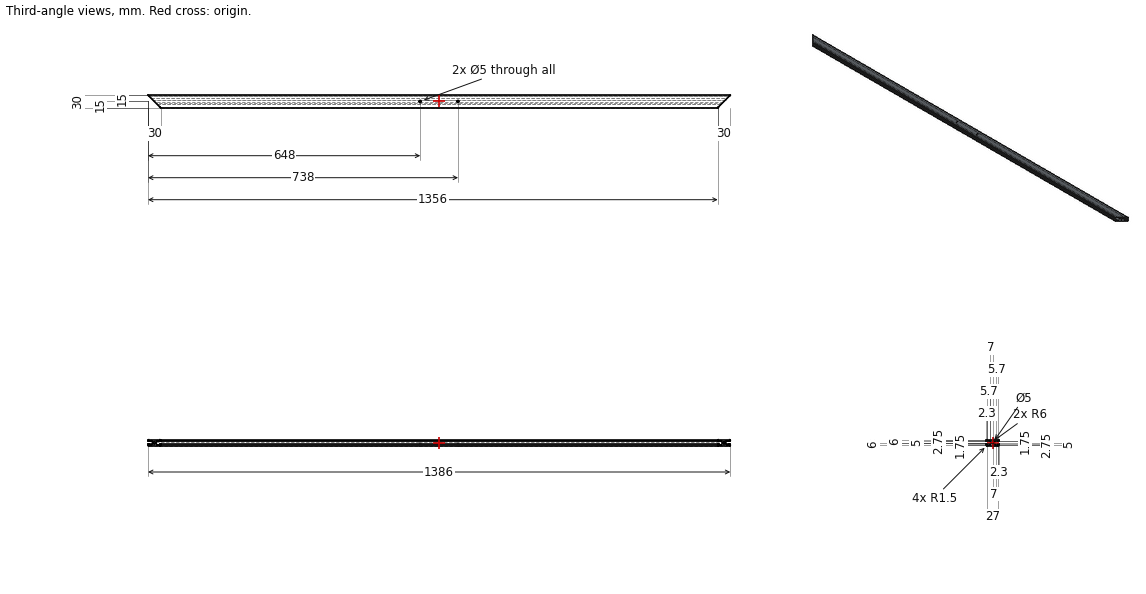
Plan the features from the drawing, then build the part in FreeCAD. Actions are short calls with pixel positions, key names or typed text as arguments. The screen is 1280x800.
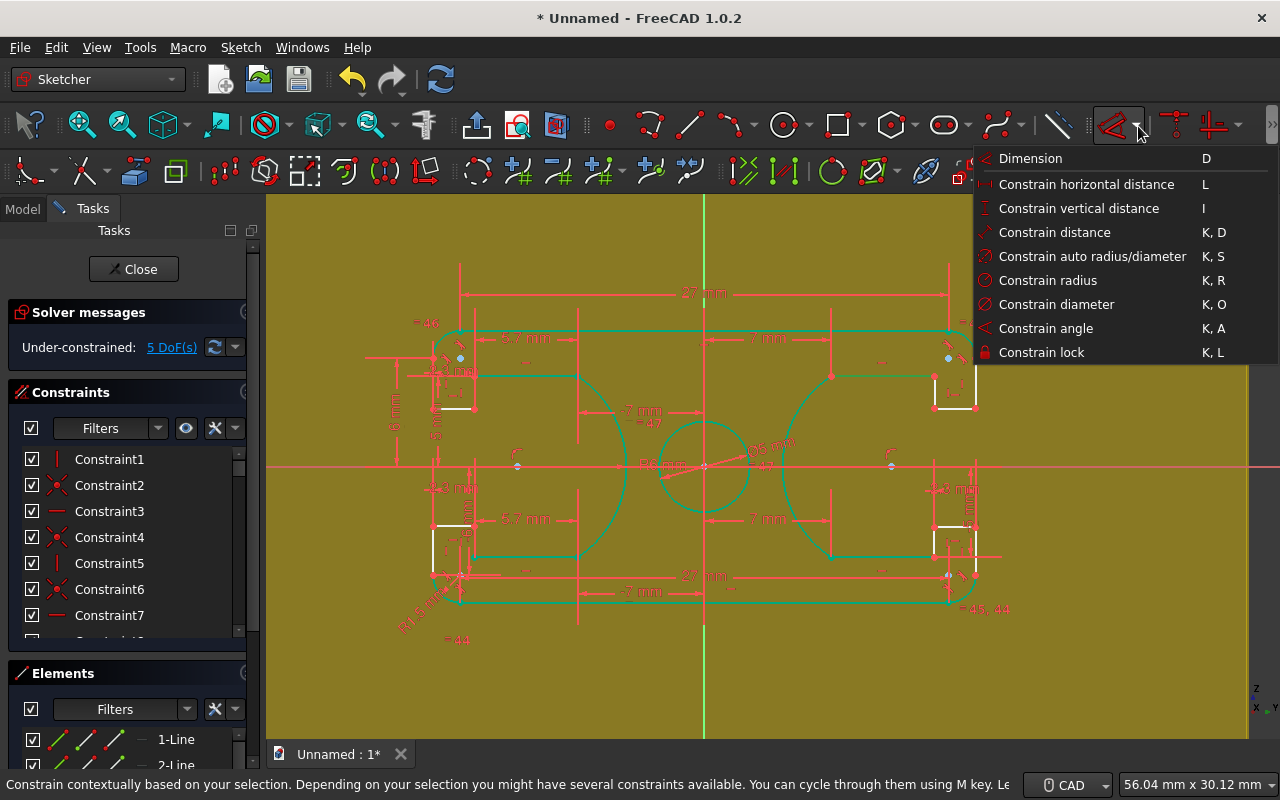
click(1126, 184)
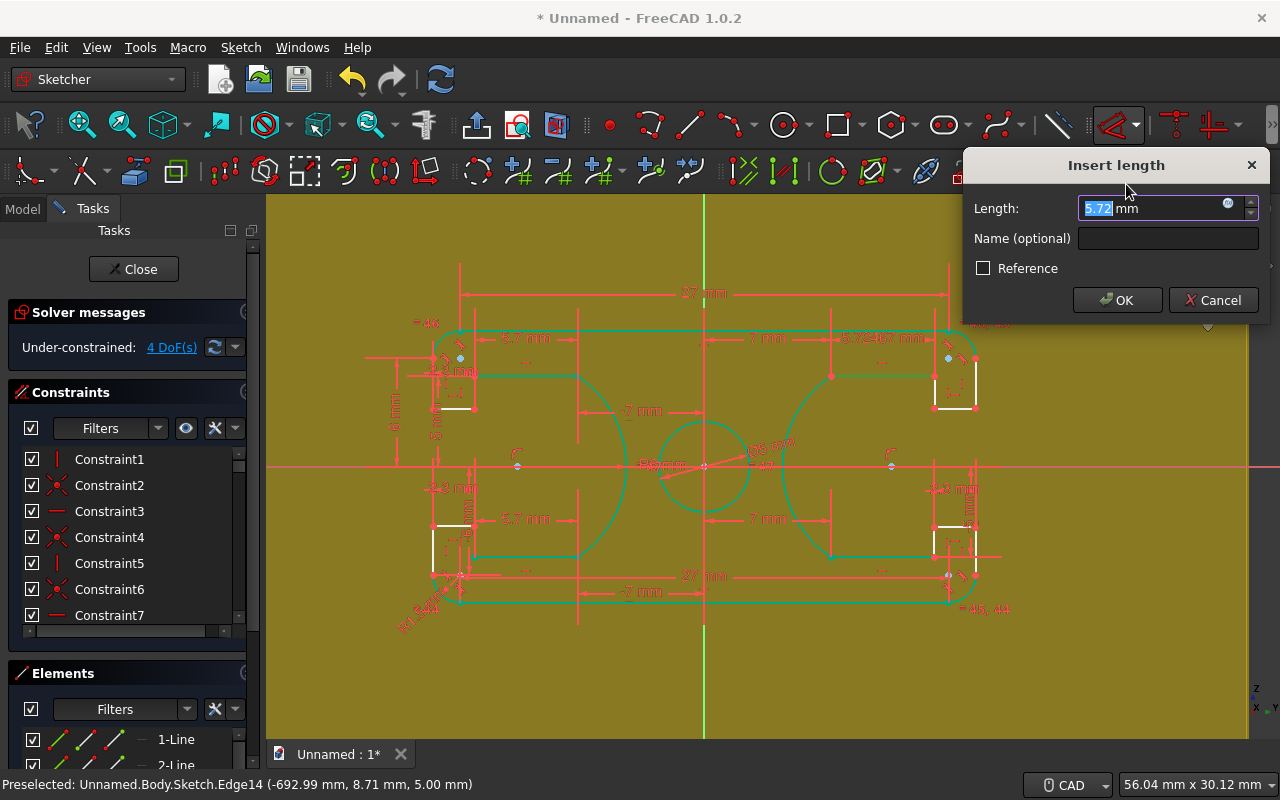
text(5.7)
key(Return)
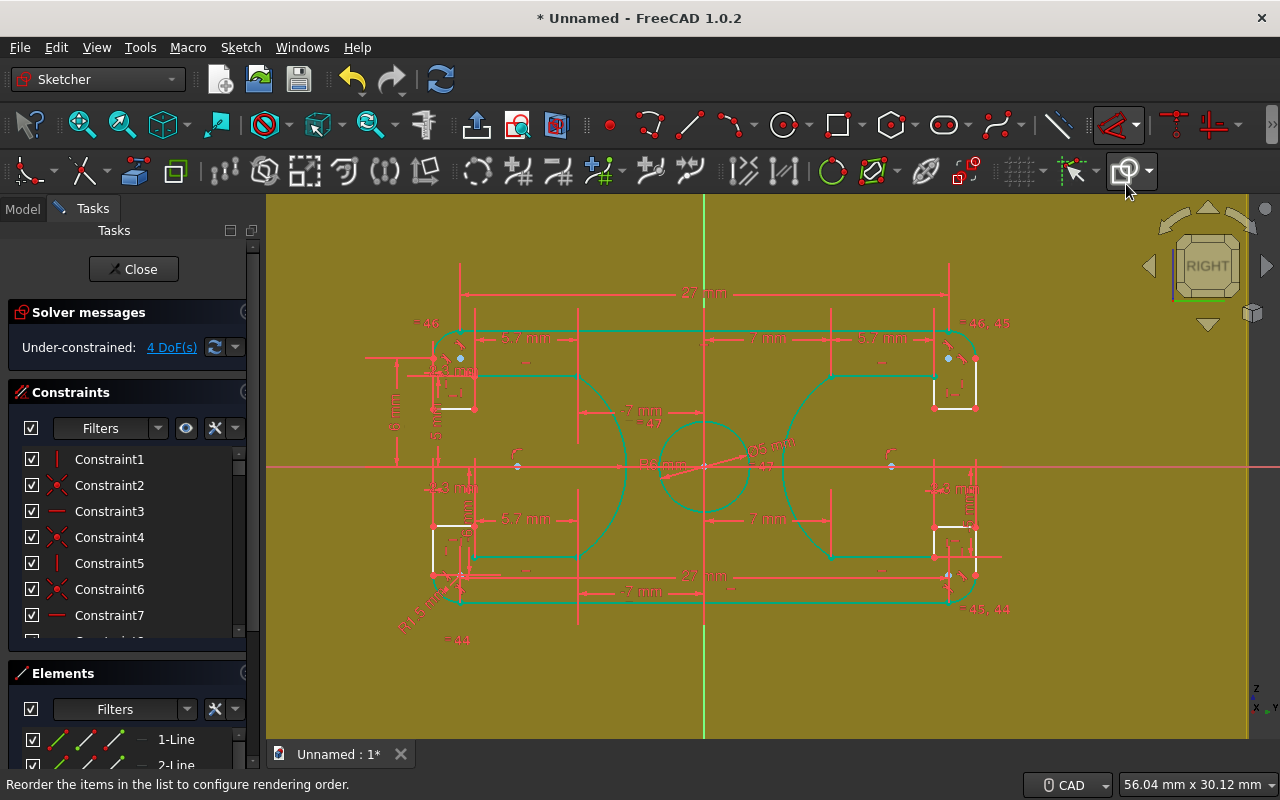
click(433, 394)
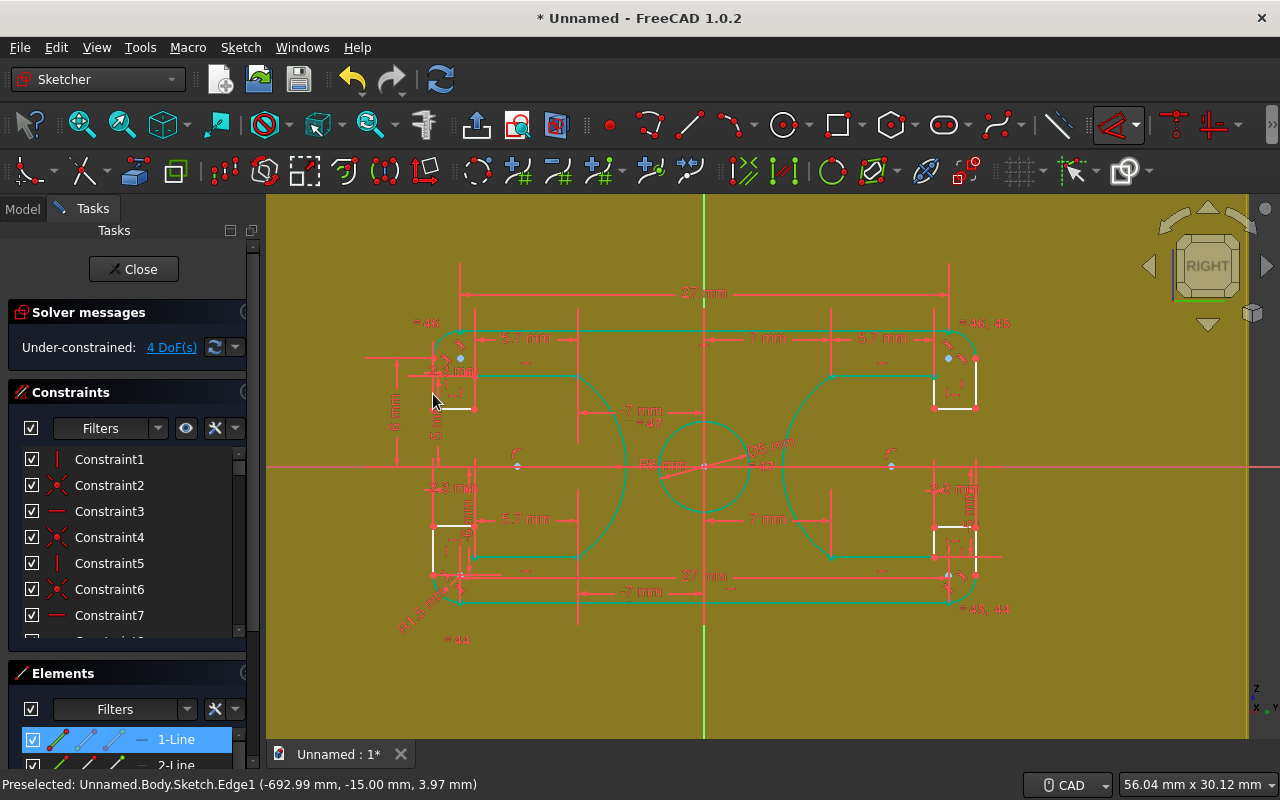
key(i)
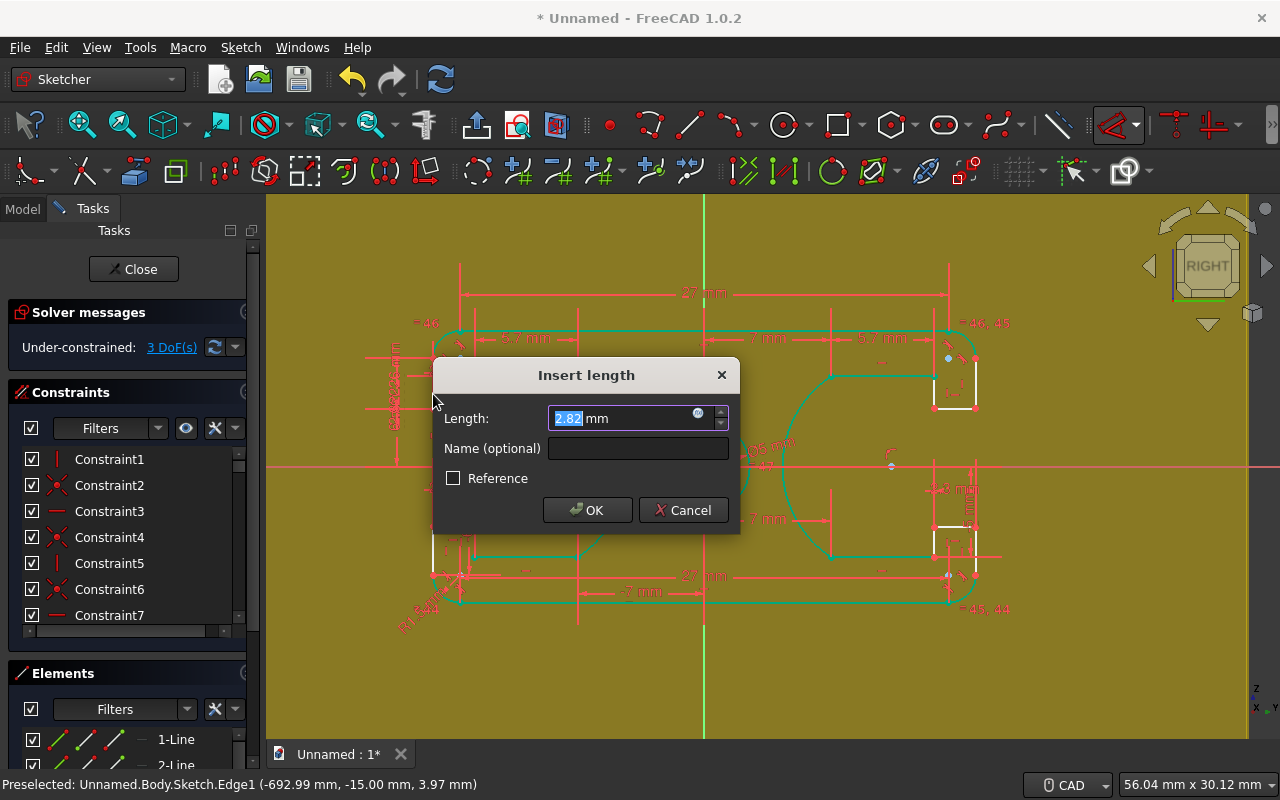
text(2.75)
key(Return)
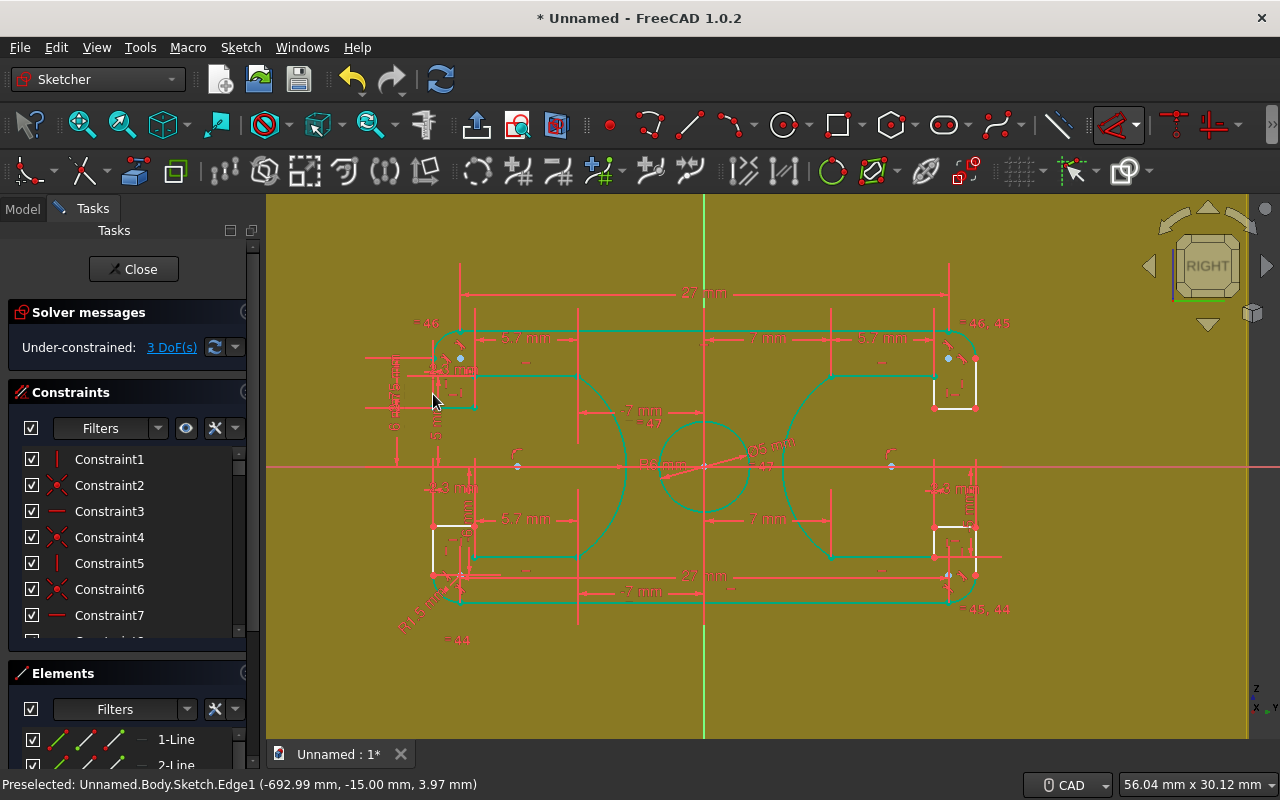
scroll(475, 548, up, 2)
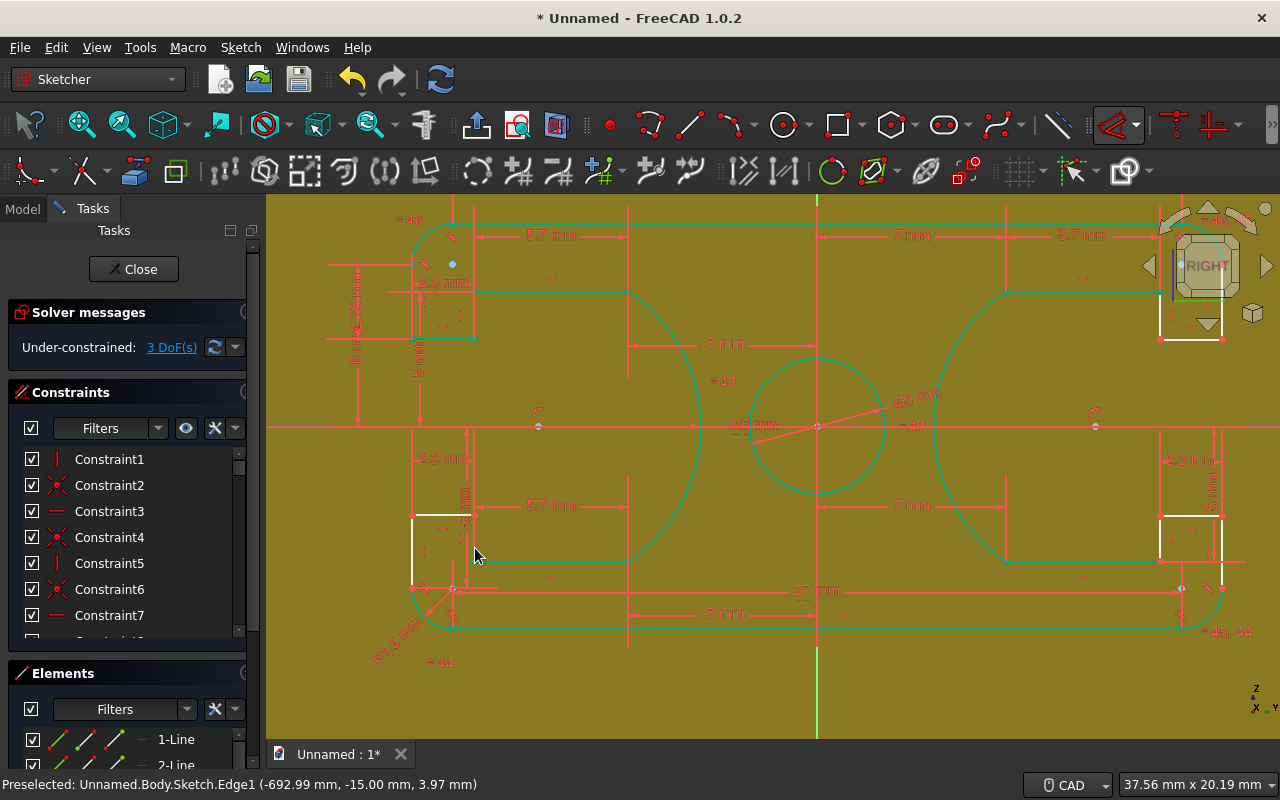
click(474, 548)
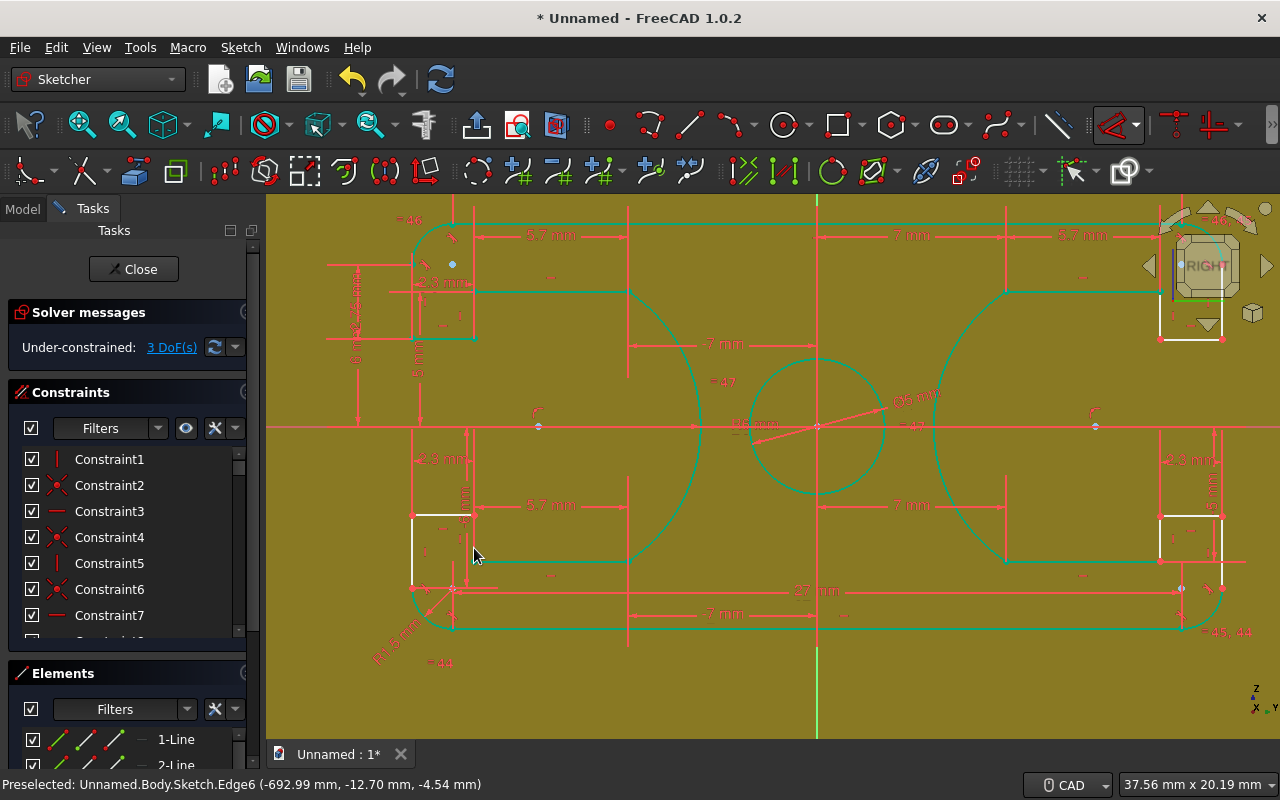
click(1138, 126)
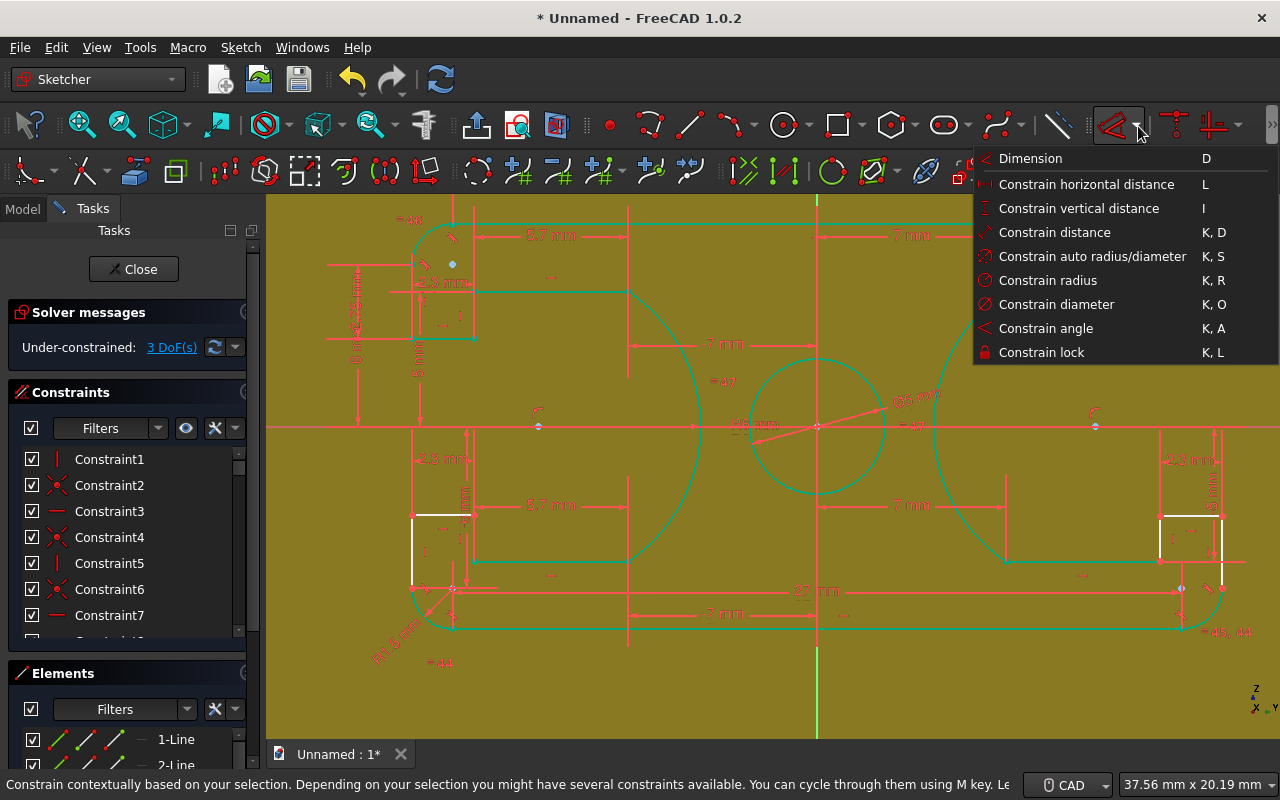
click(1126, 208)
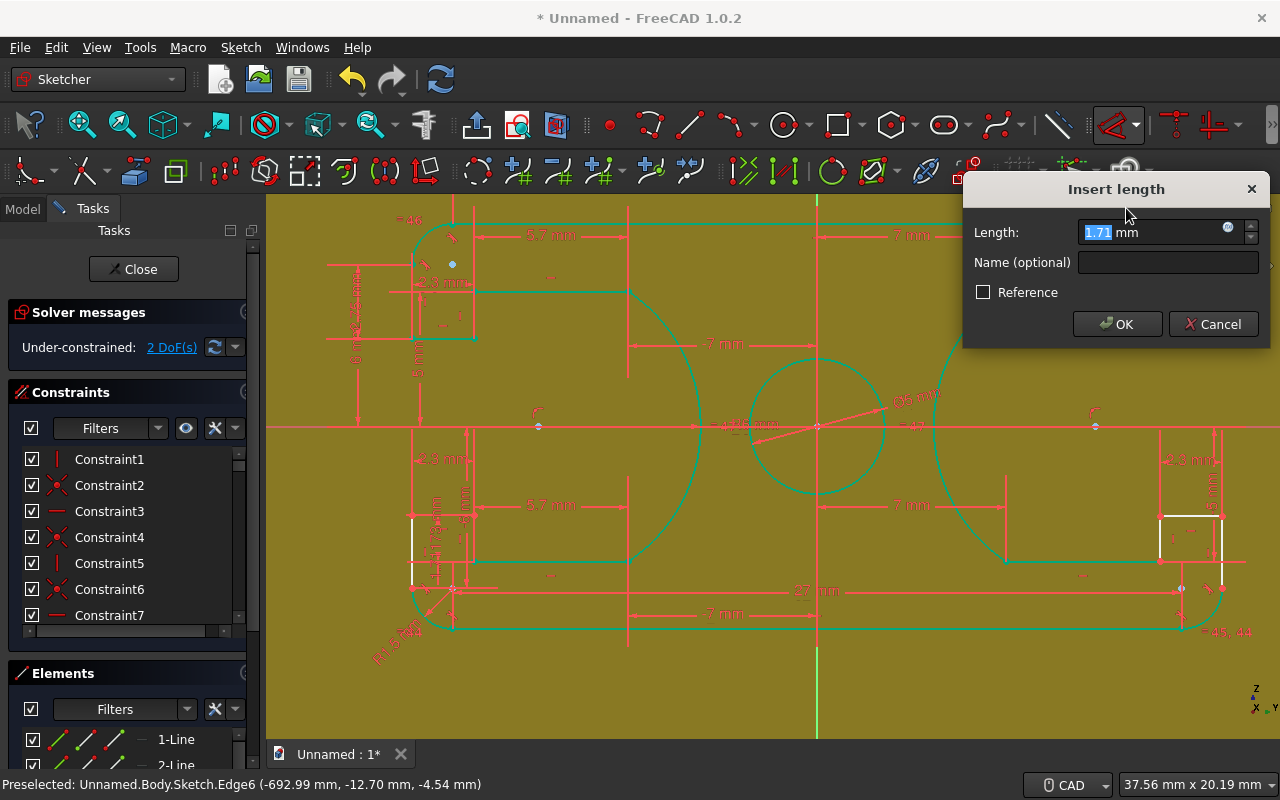
text(1.75)
key(Return)